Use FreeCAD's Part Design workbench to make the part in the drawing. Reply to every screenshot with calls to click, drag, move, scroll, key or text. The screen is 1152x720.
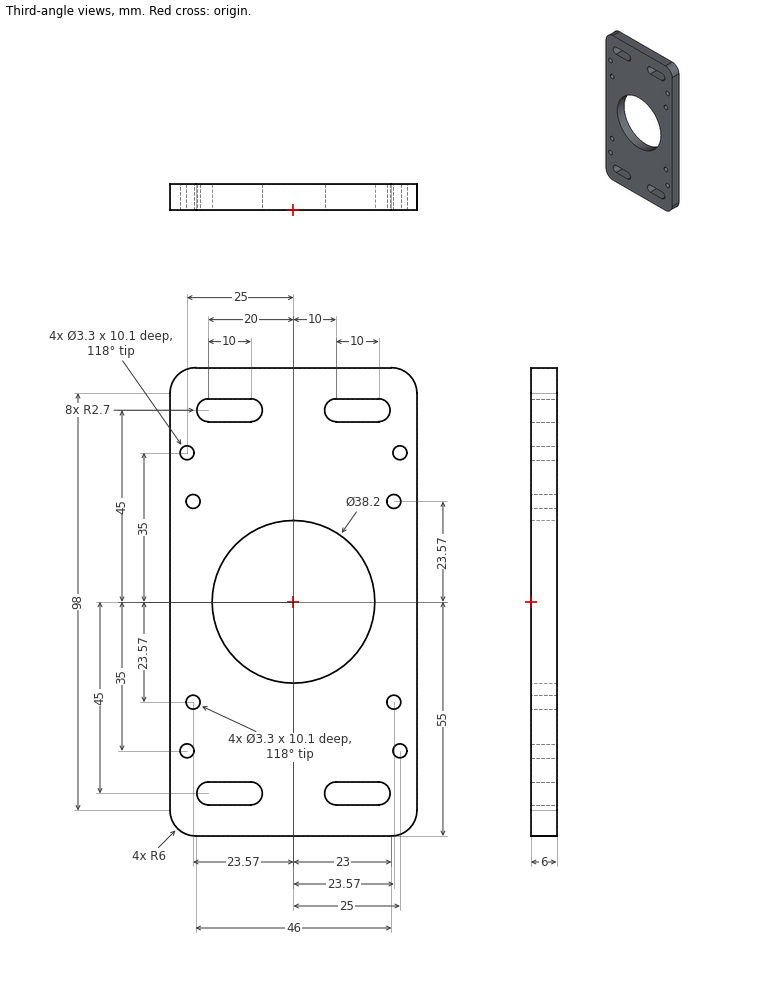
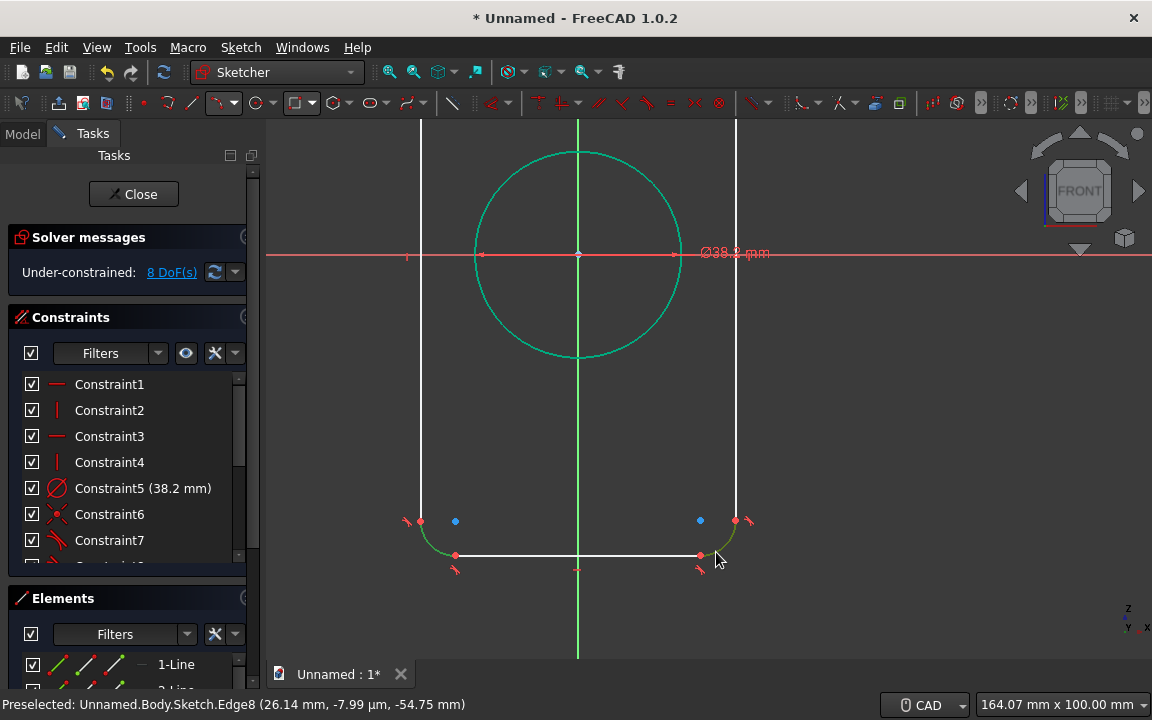
key(e)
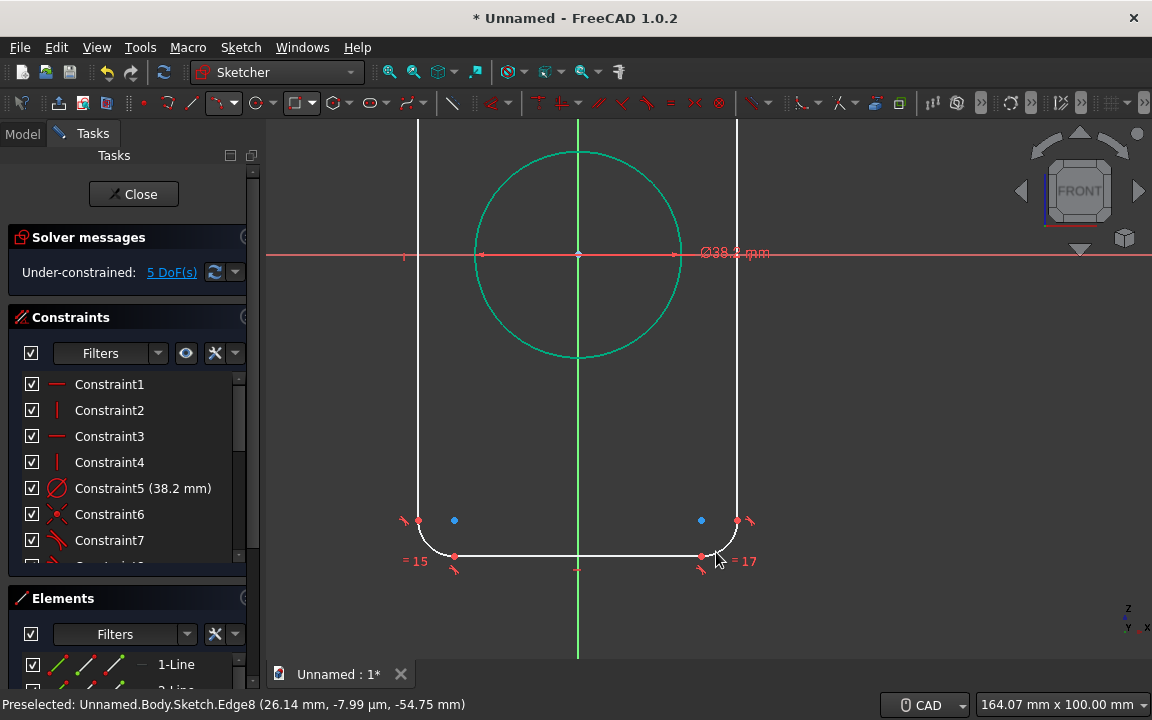
scroll(422, 537, up, 2)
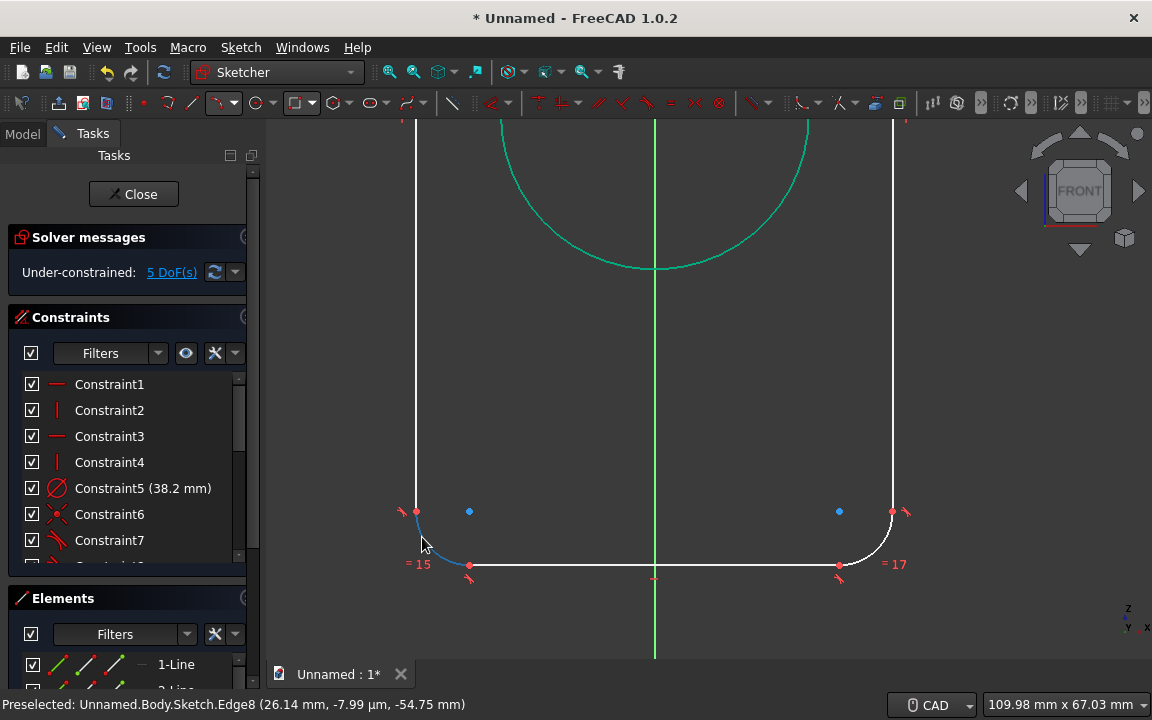
click(422, 536)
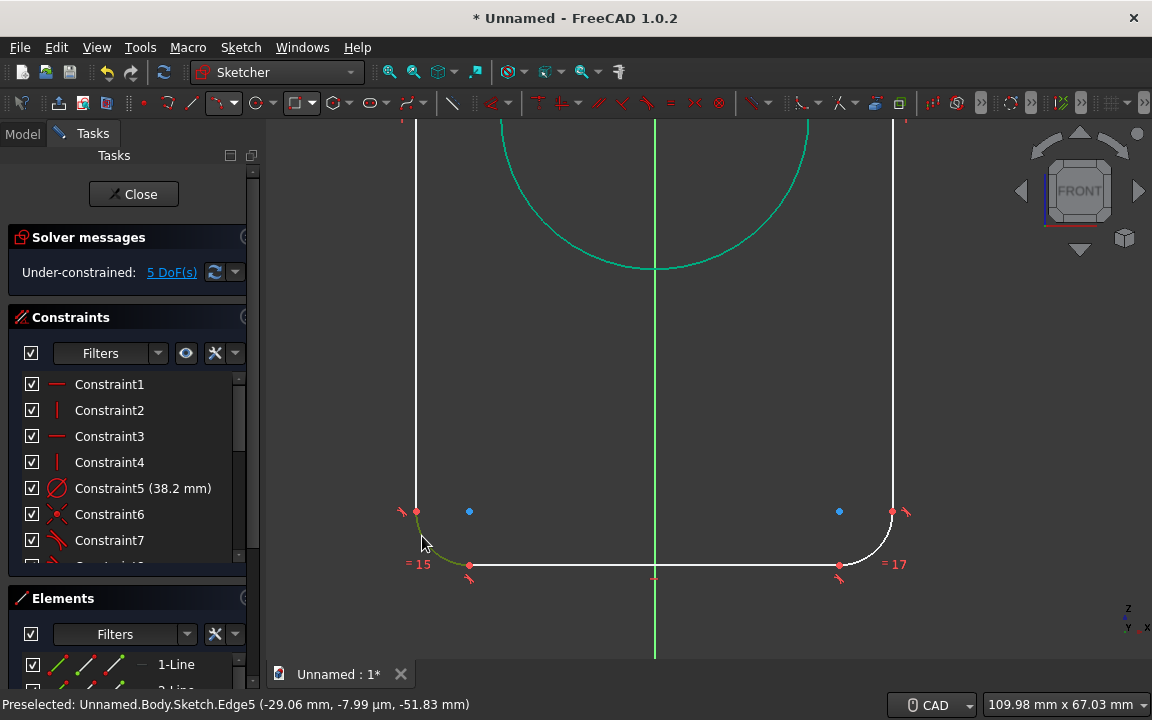
click(510, 104)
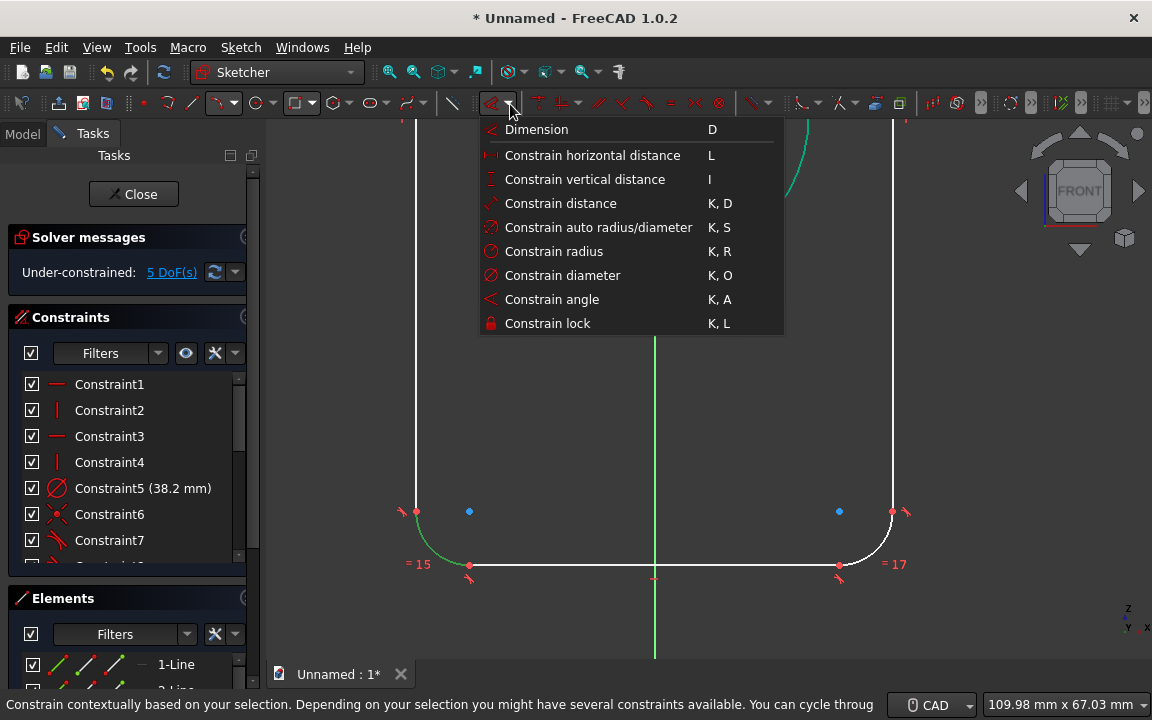
click(632, 251)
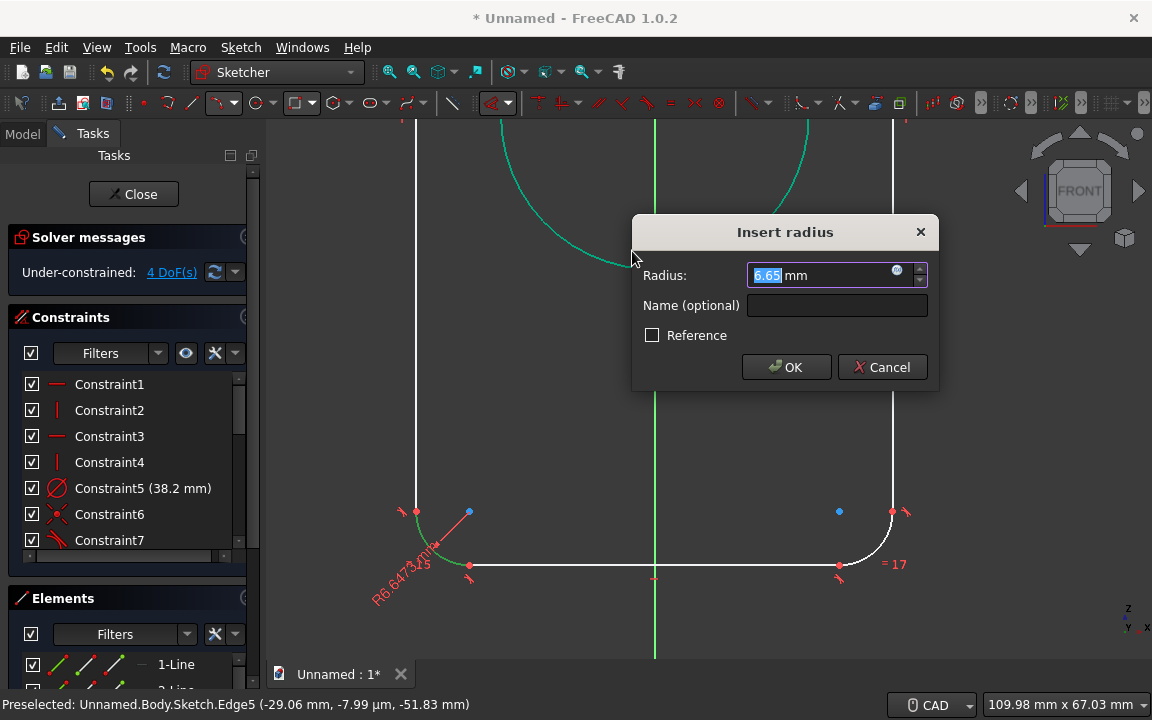
text(6)
key(Return)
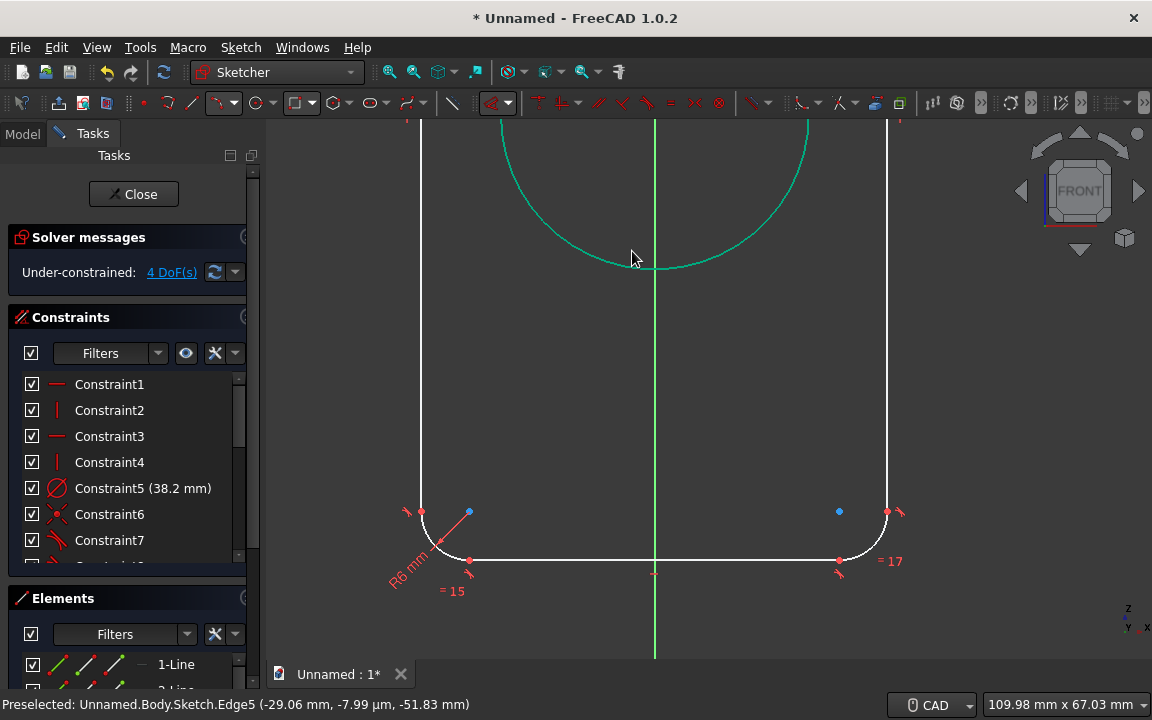
click(728, 560)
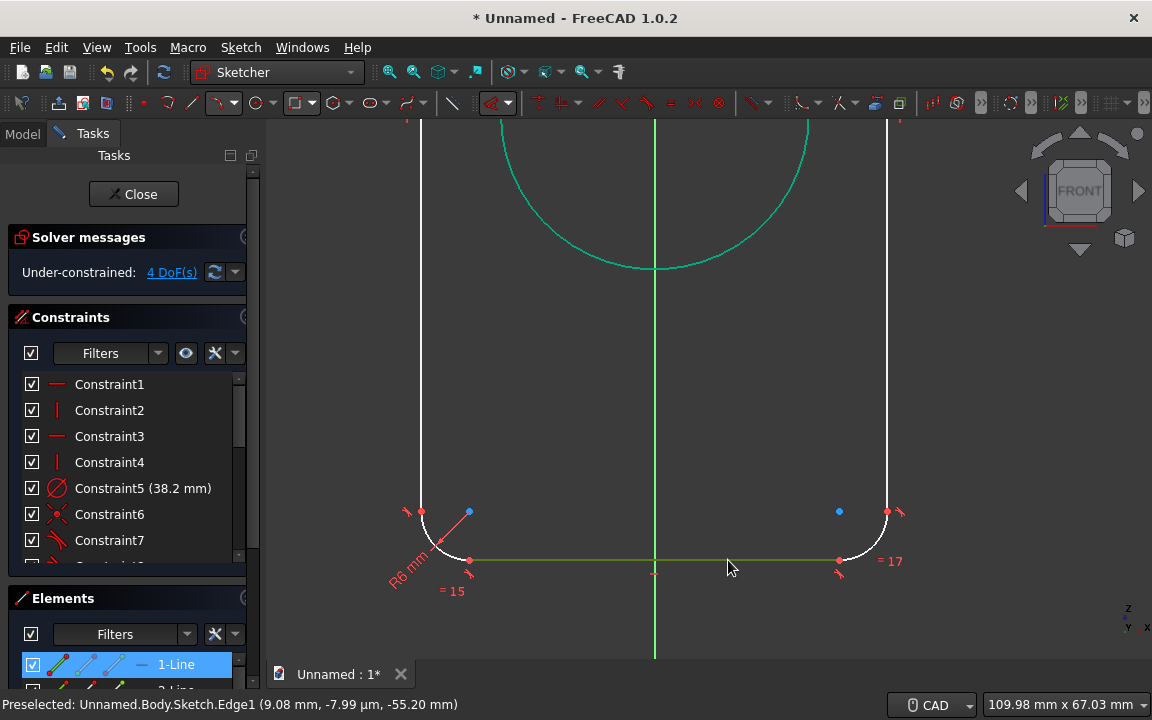
click(510, 104)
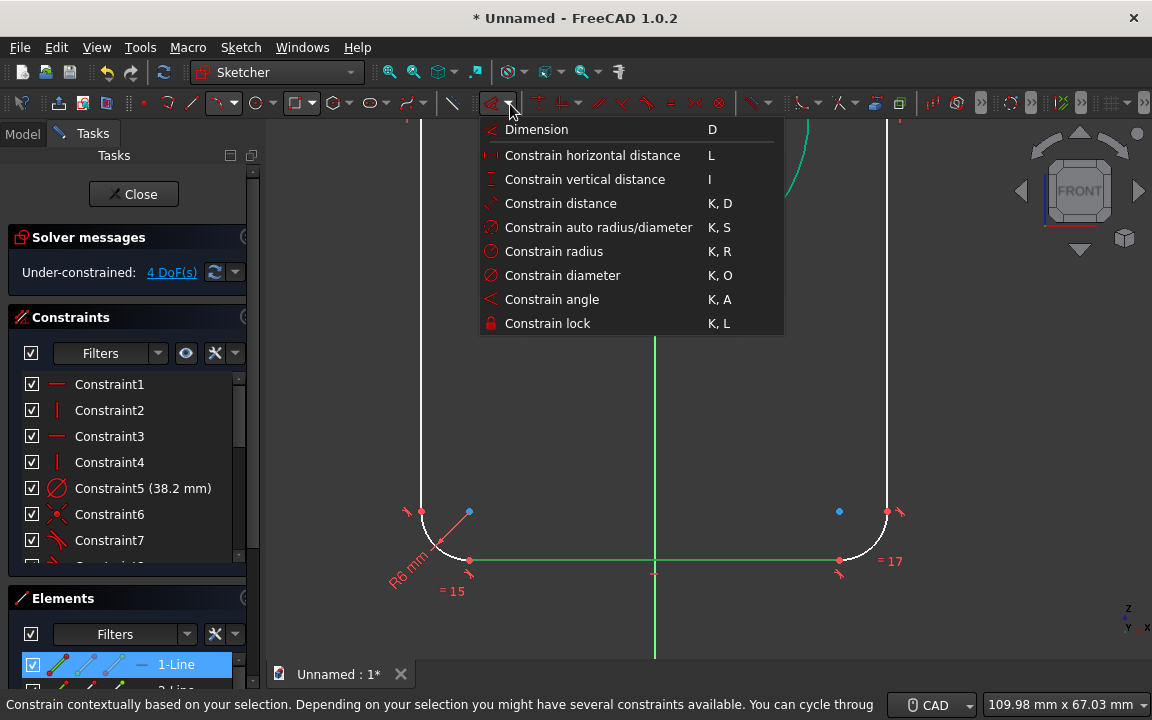
click(632, 155)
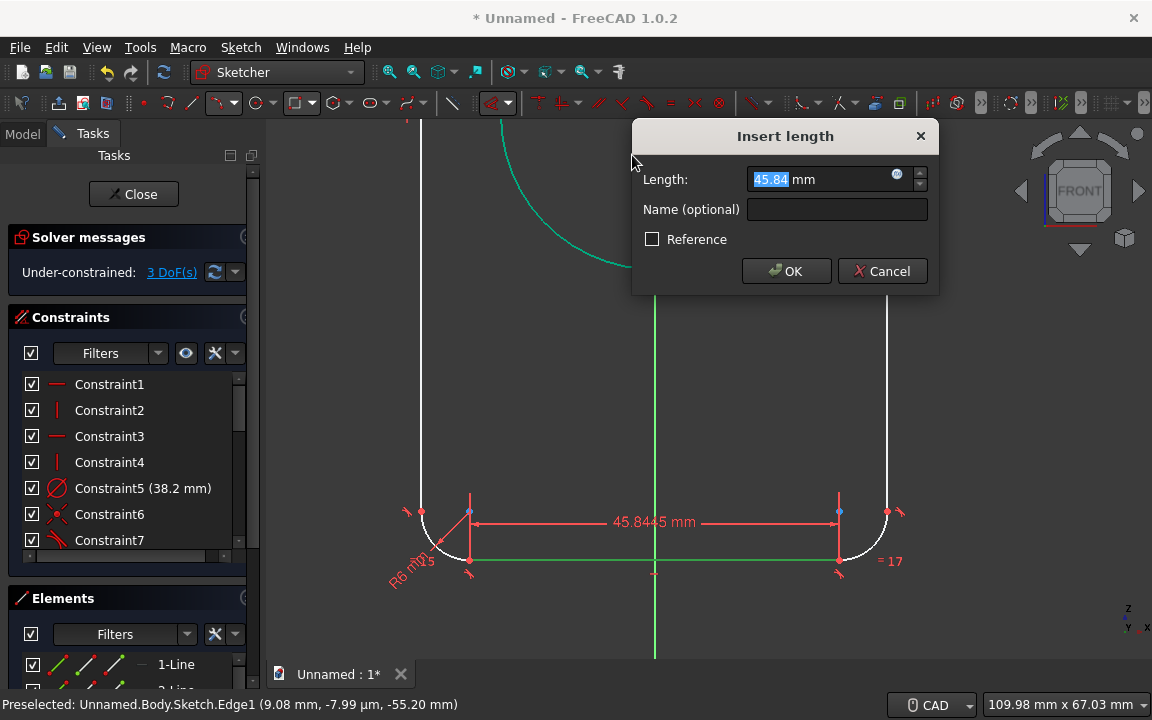
text(46)
key(Return)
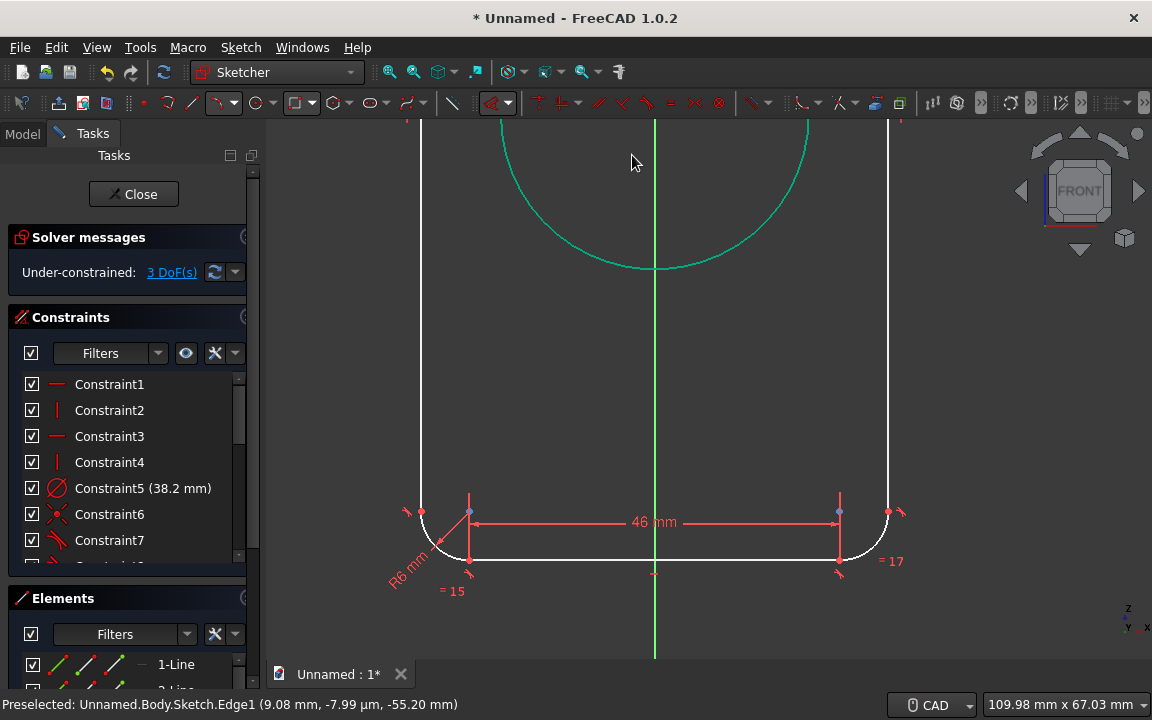
click(421, 276)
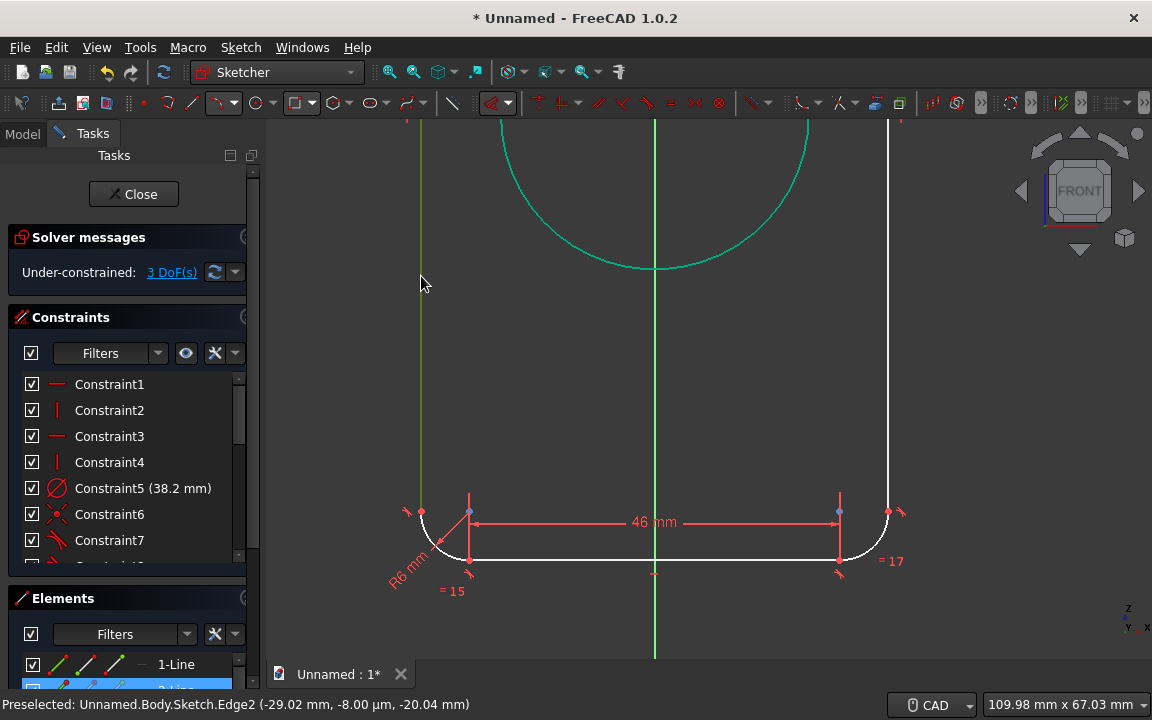
click(510, 104)